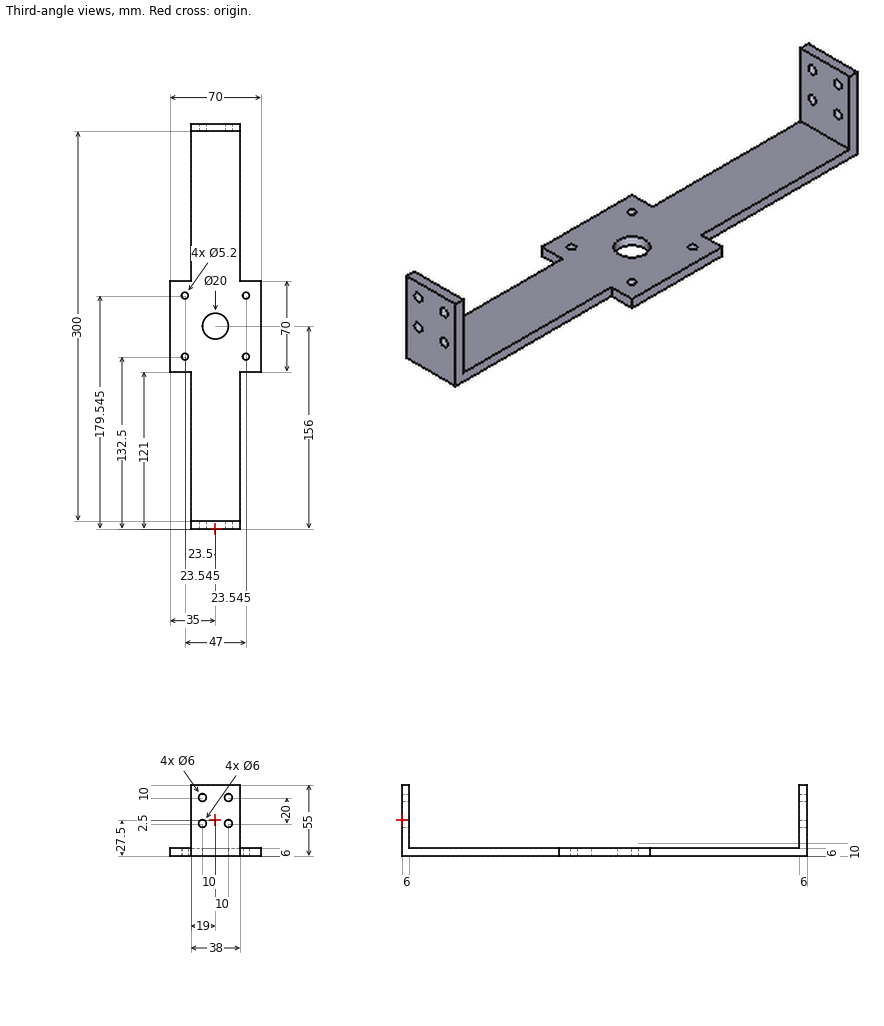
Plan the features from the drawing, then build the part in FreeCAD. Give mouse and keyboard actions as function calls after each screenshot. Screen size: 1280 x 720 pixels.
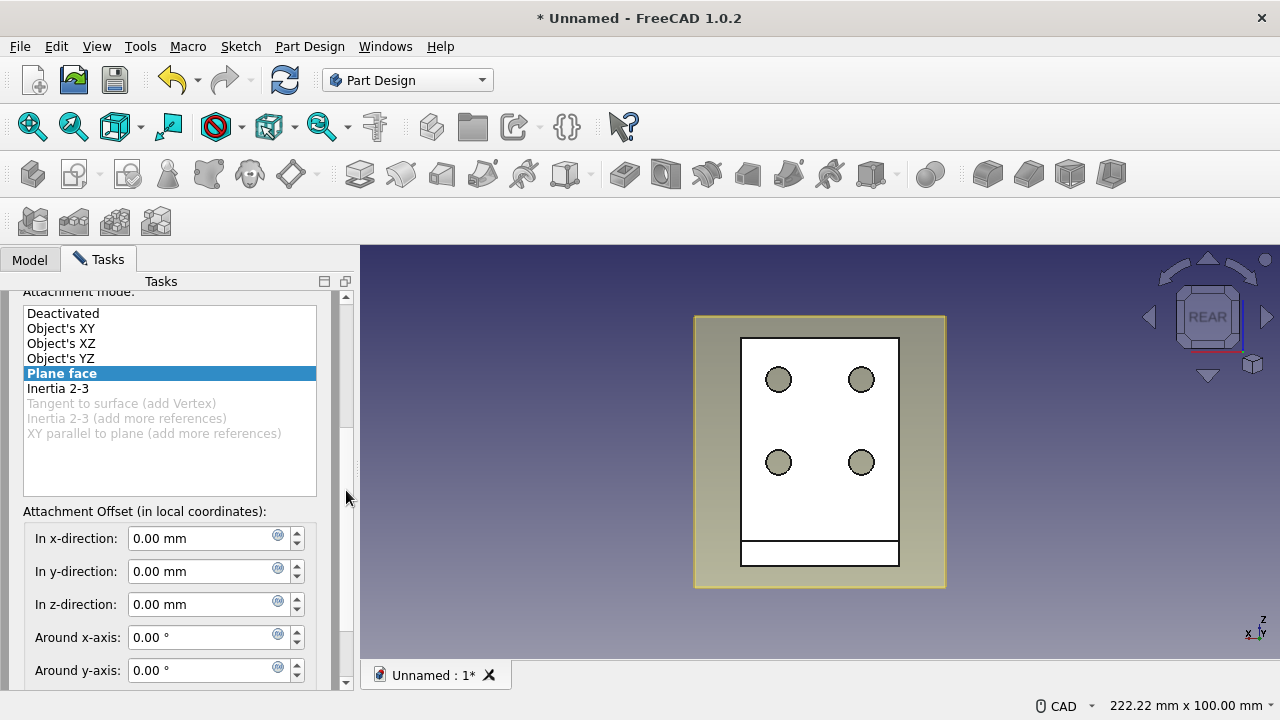
triple_click(210, 604)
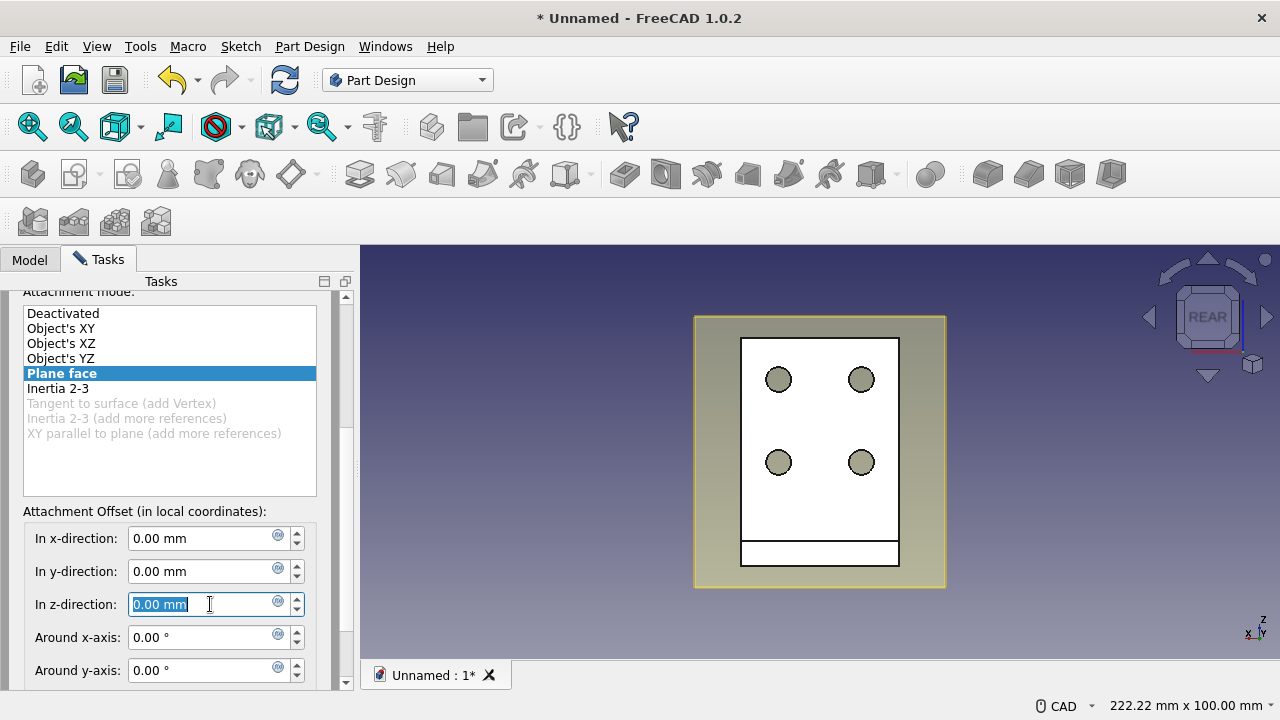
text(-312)
key(Tab)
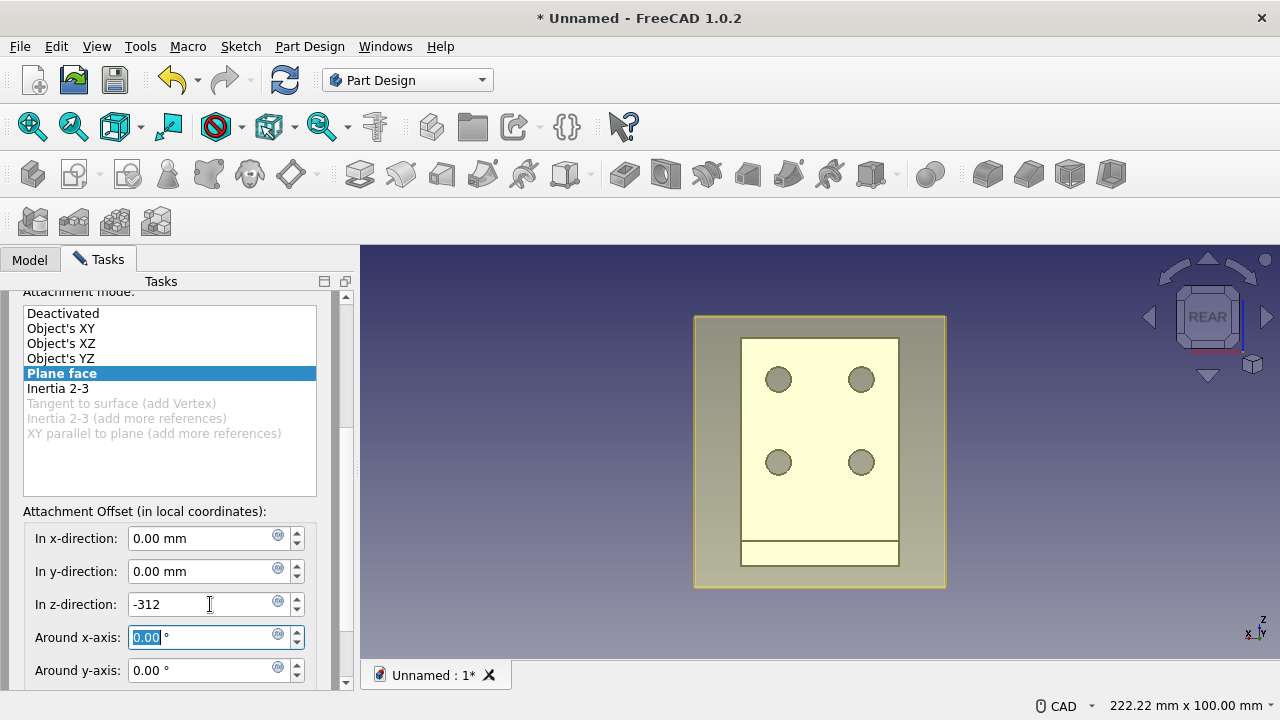
scroll(346, 490, up, 5)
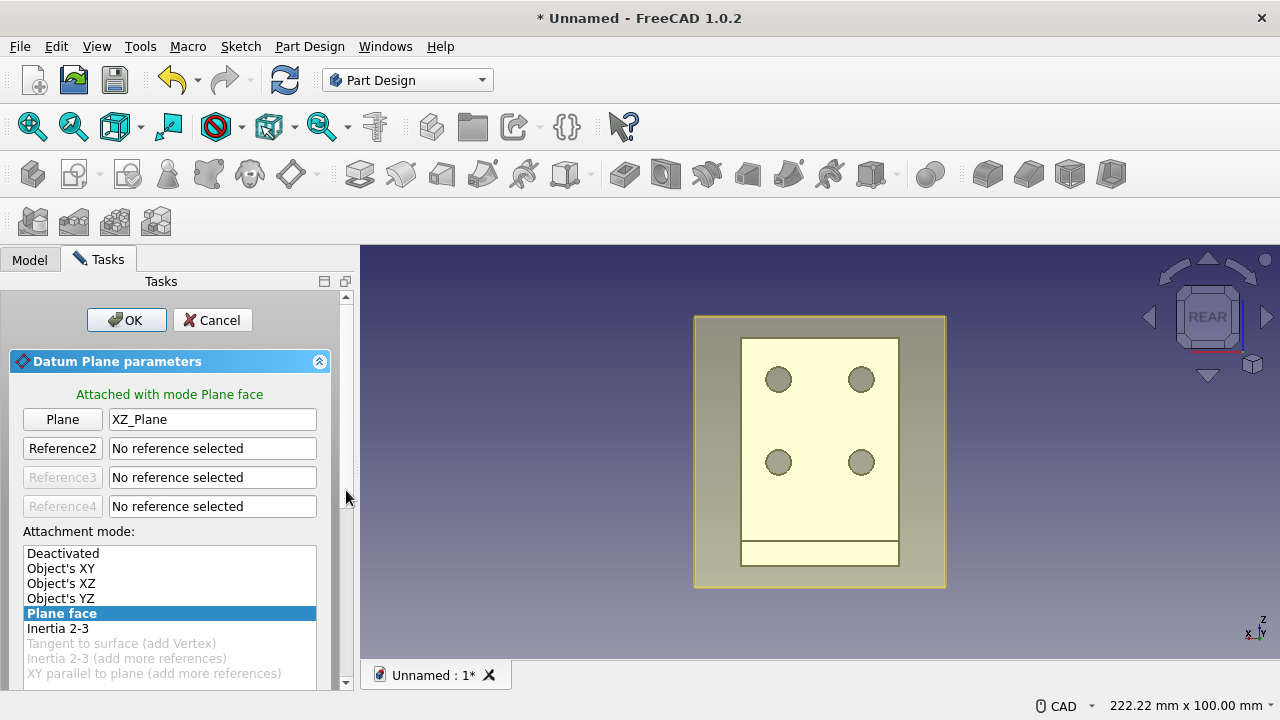
click(127, 320)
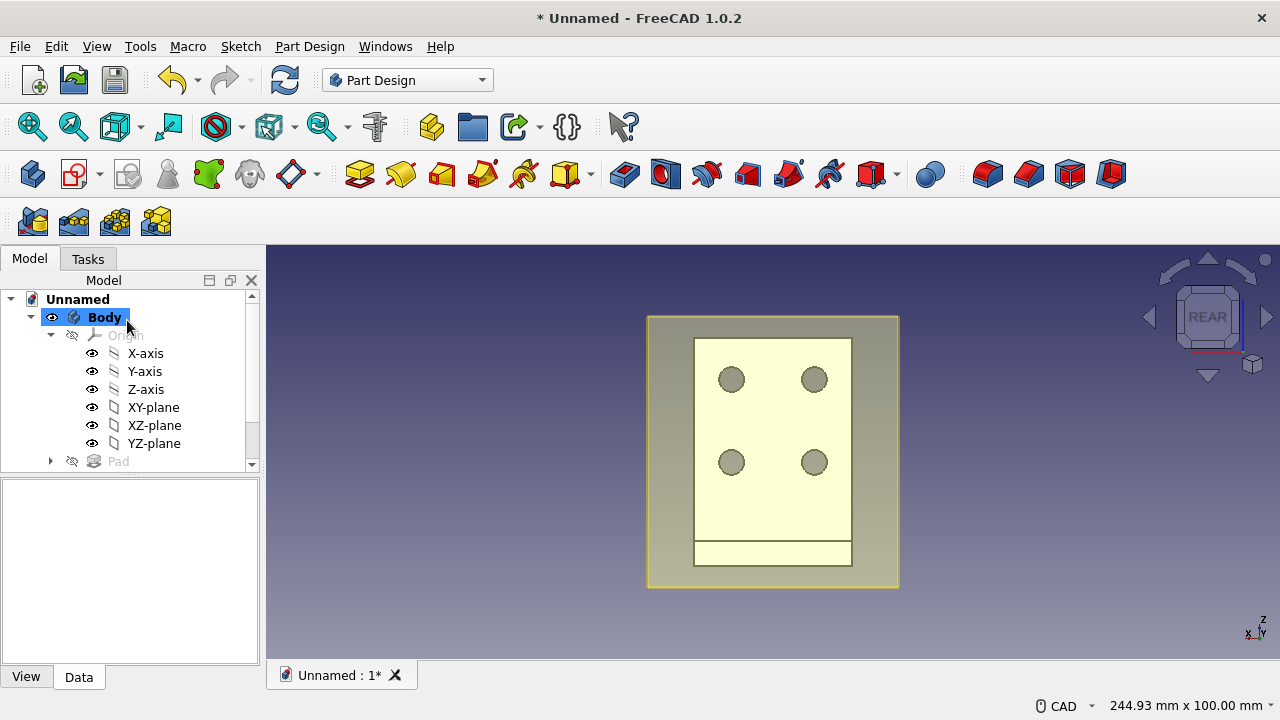
scroll(101, 385, down, 3)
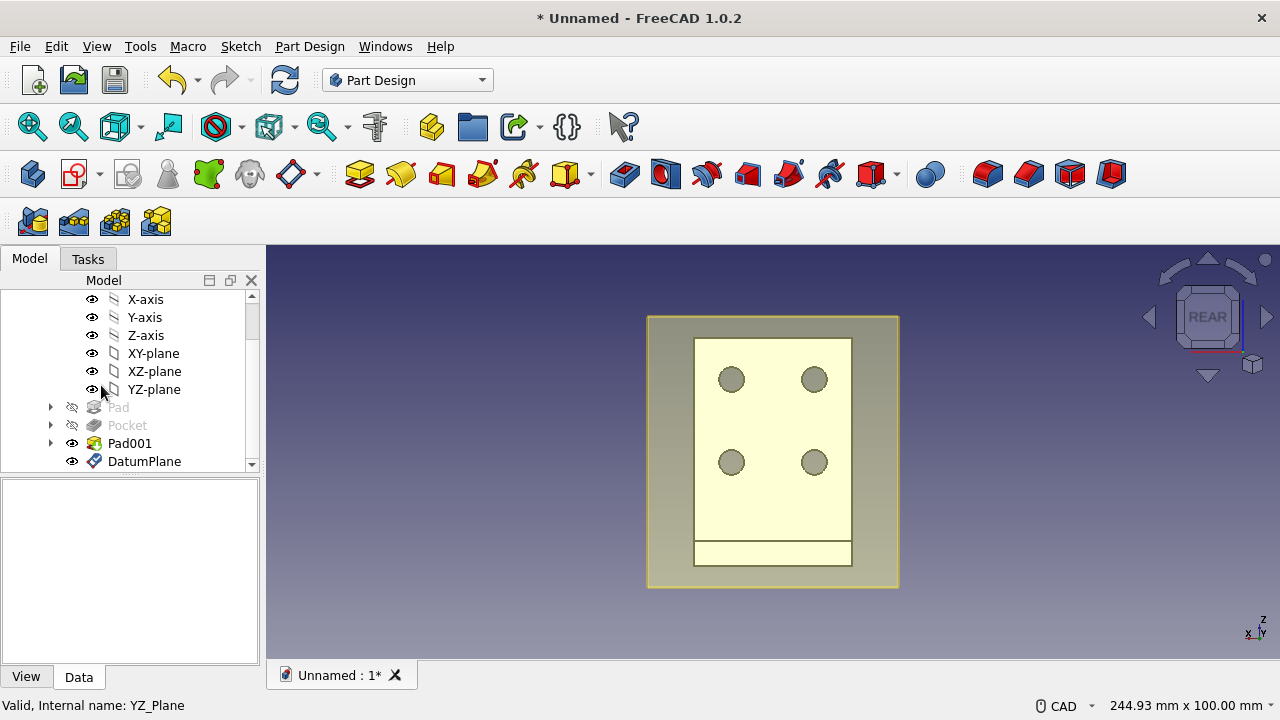
click(117, 461)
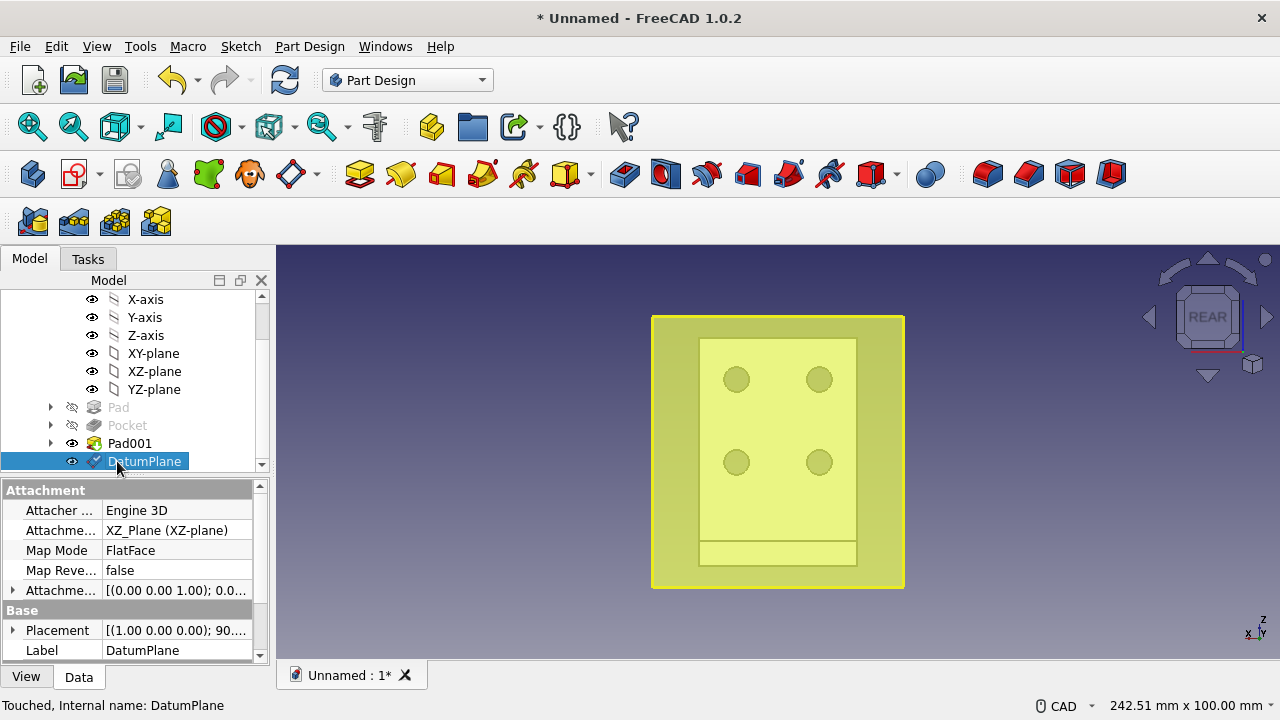
click(74, 174)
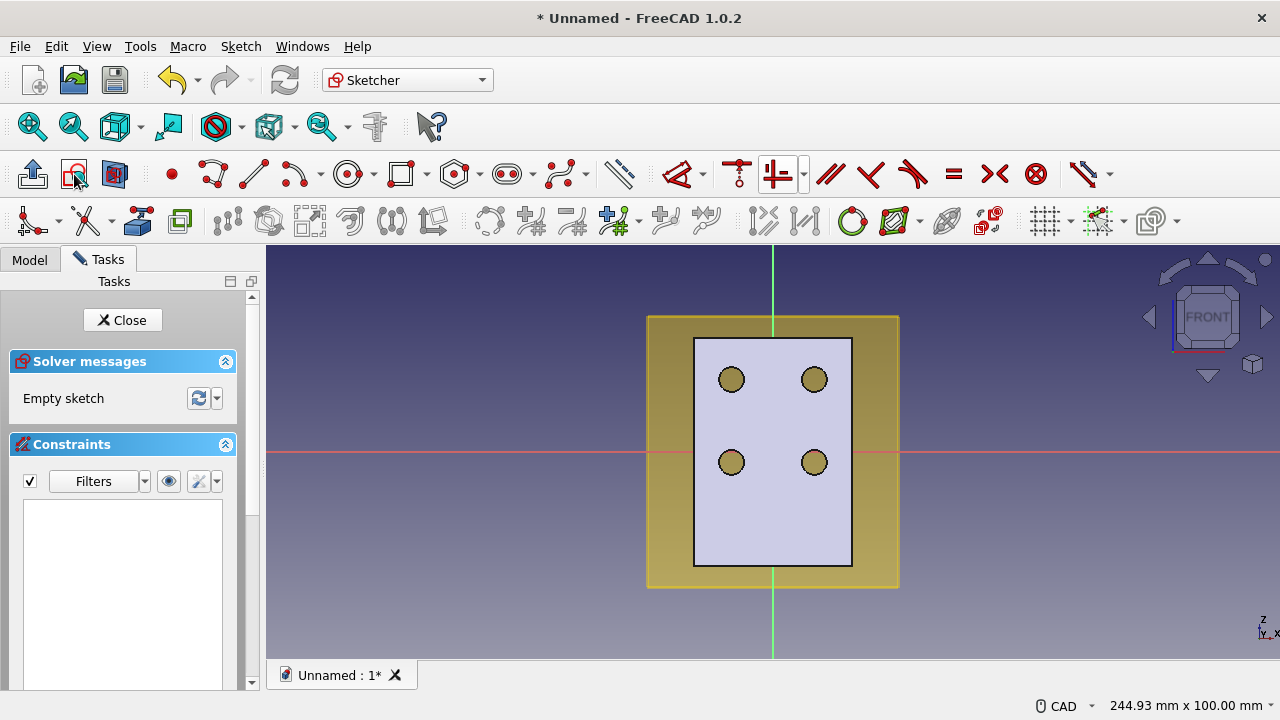
click(115, 174)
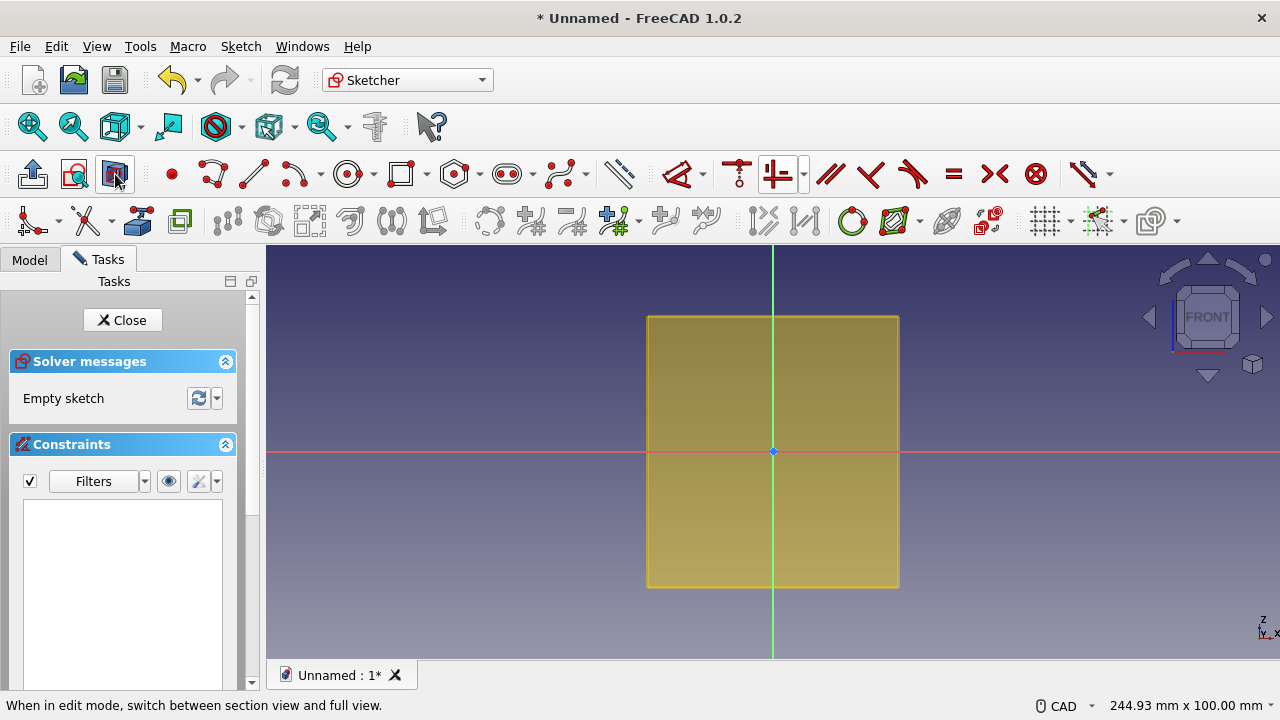
click(426, 174)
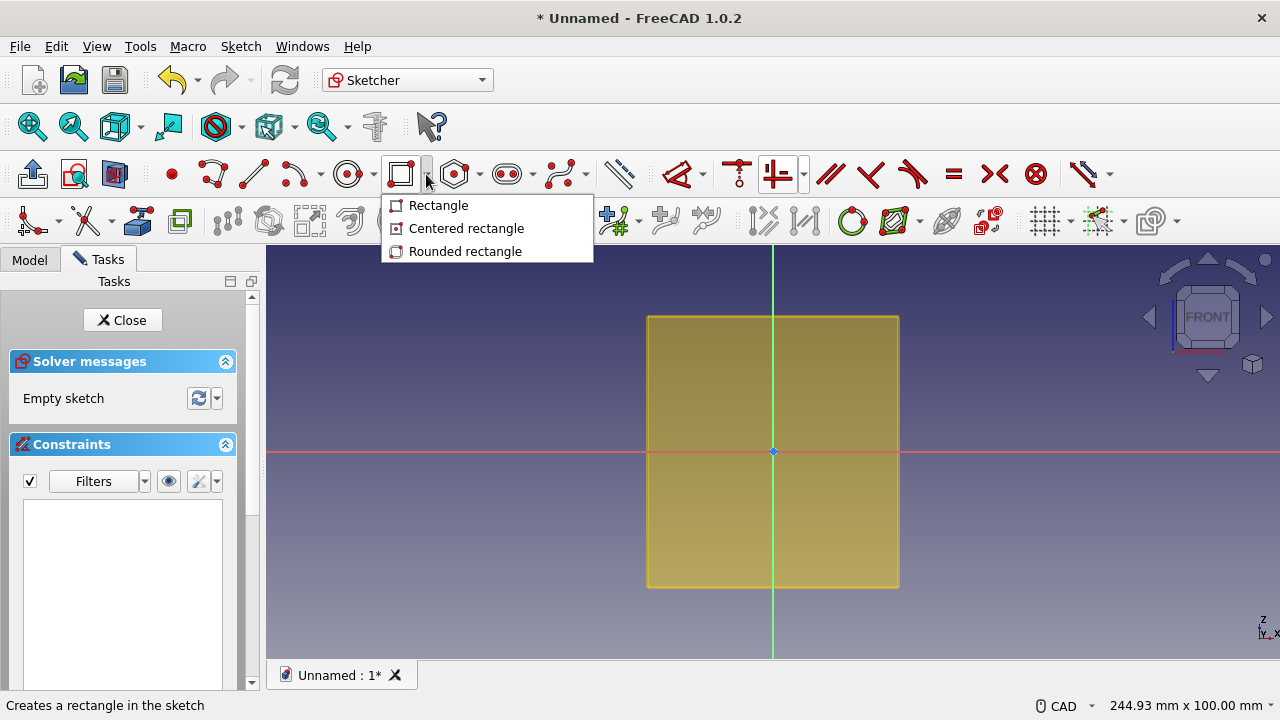
click(488, 228)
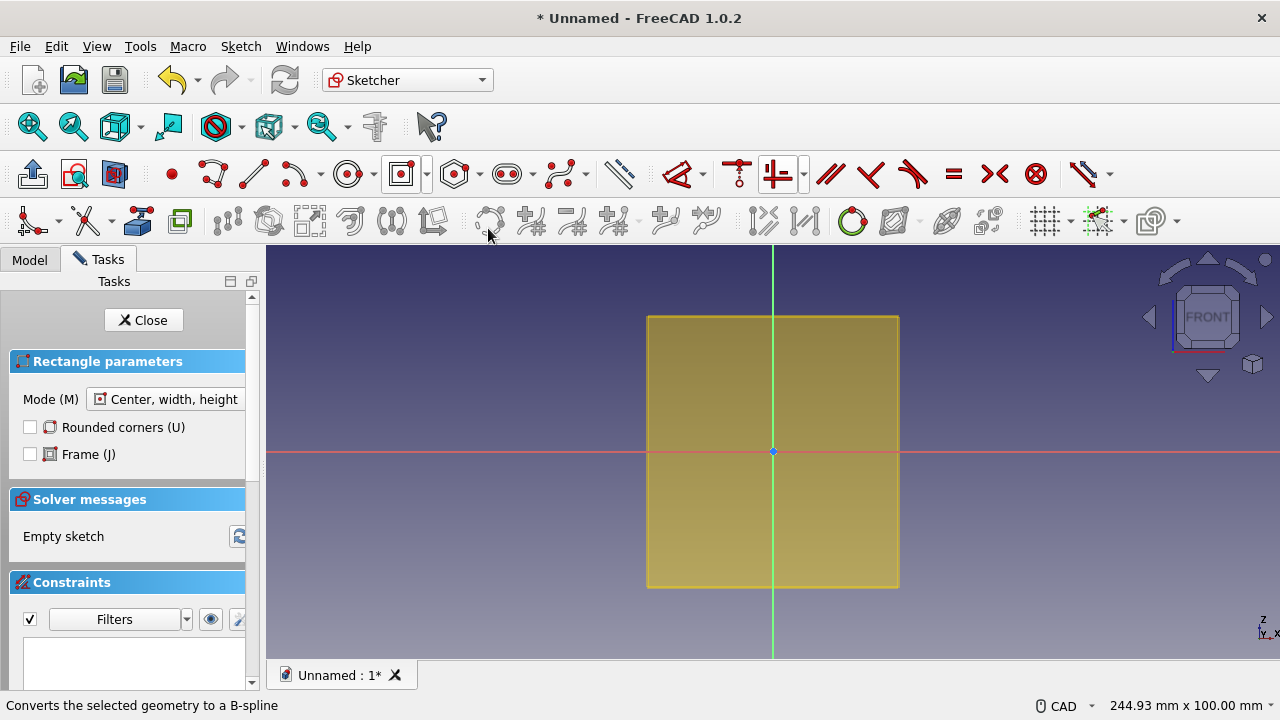
click(773, 452)
move(852, 338)